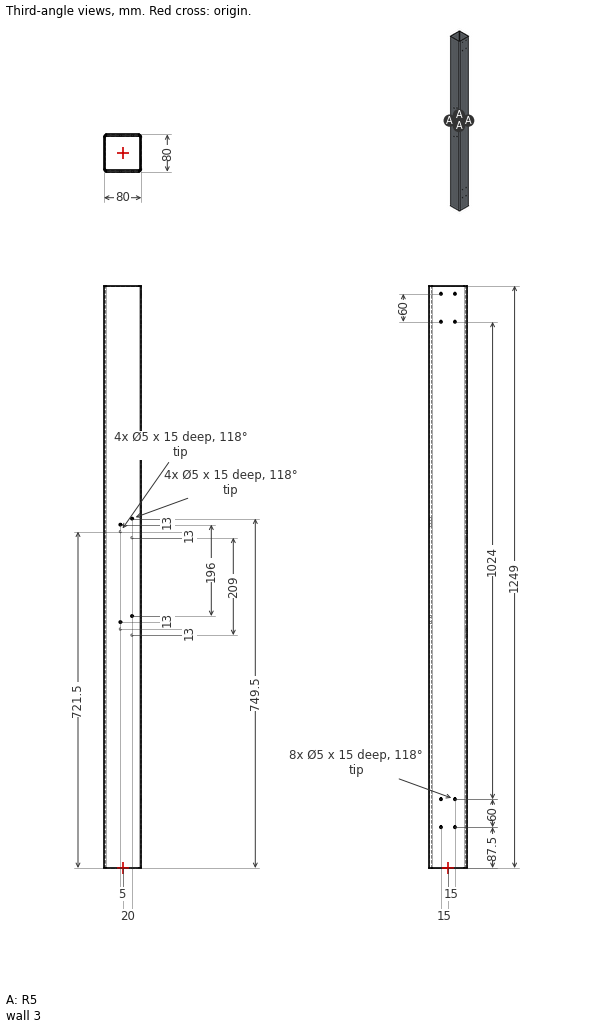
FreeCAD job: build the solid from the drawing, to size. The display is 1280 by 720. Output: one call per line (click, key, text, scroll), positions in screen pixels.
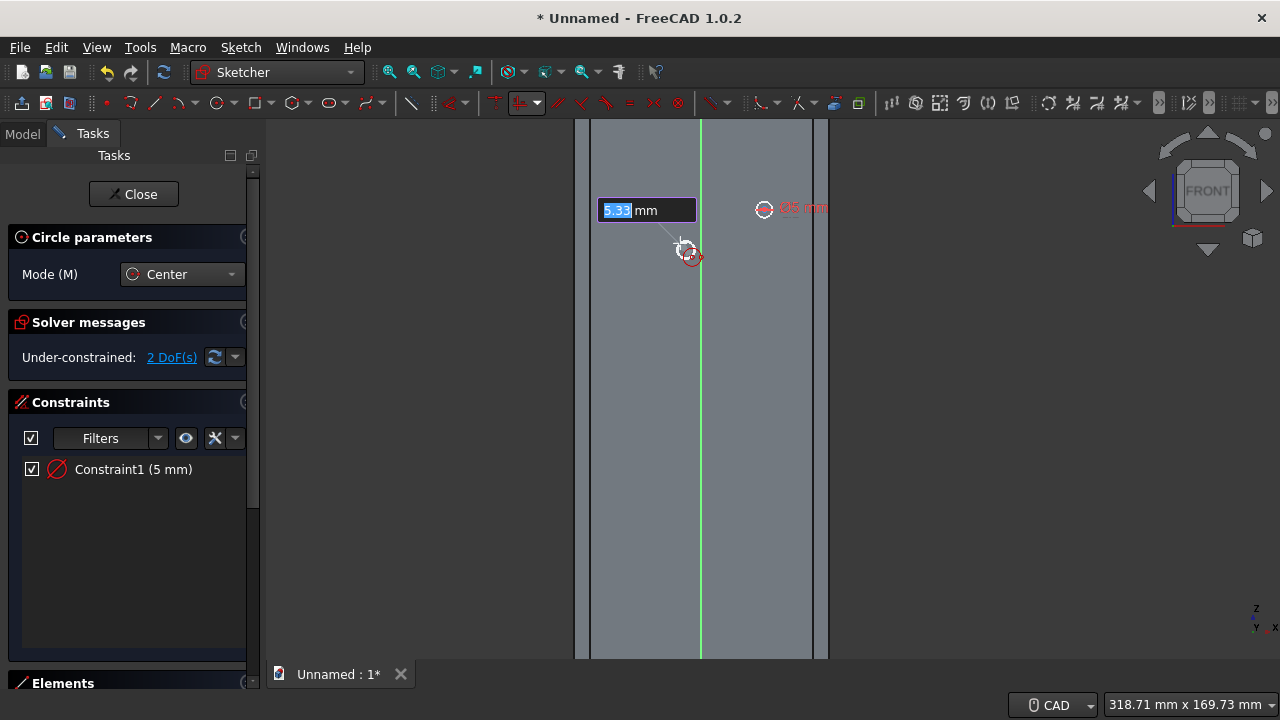
text(5)
key(Return)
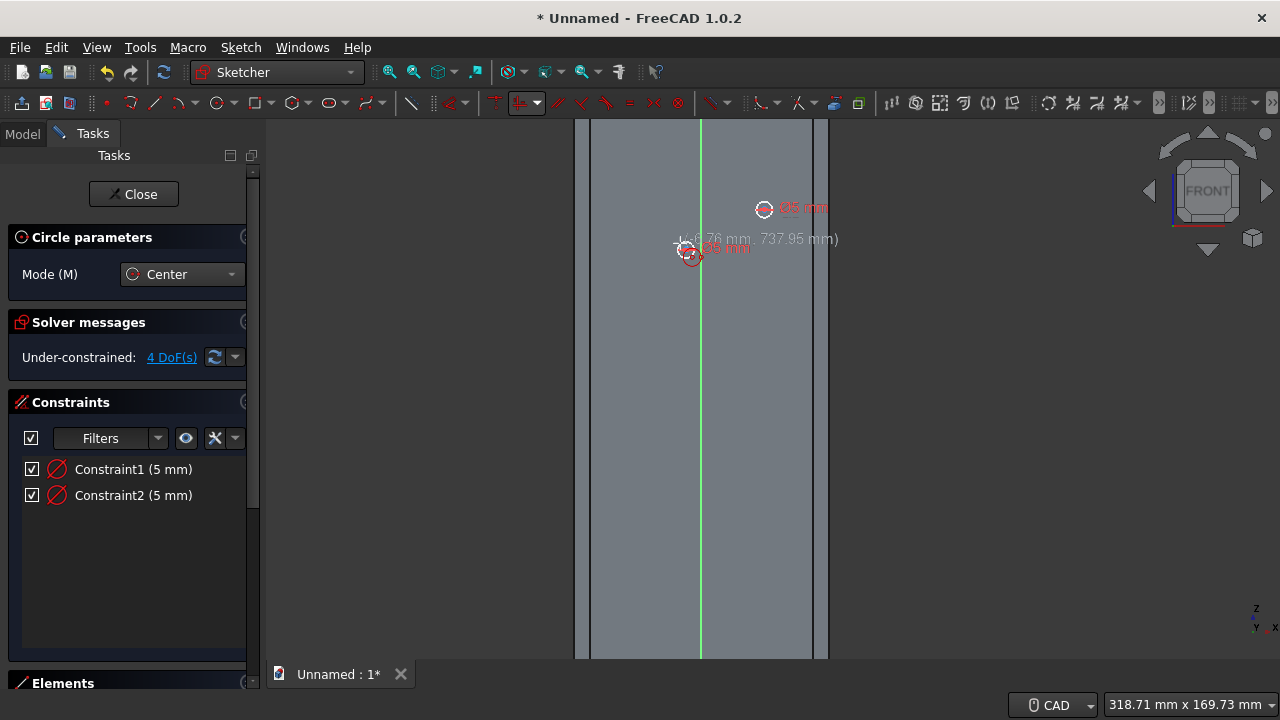
scroll(687, 249, down, 4)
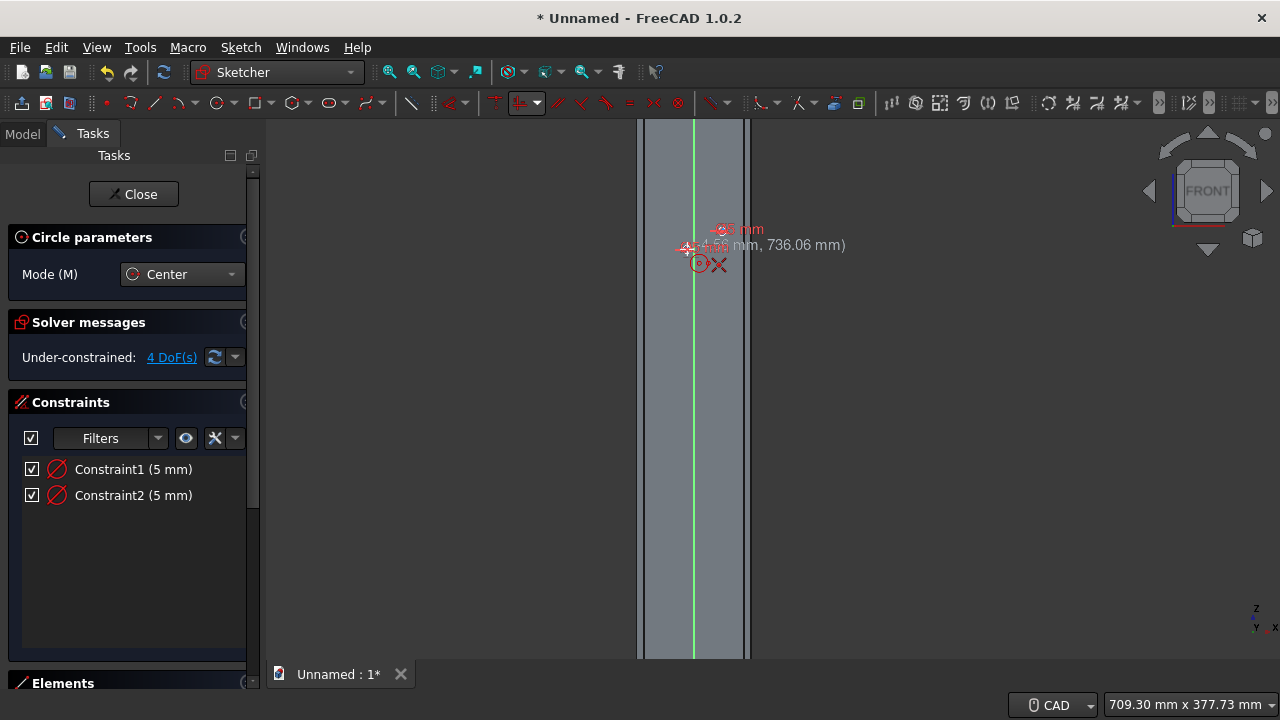
scroll(722, 529, up, 10)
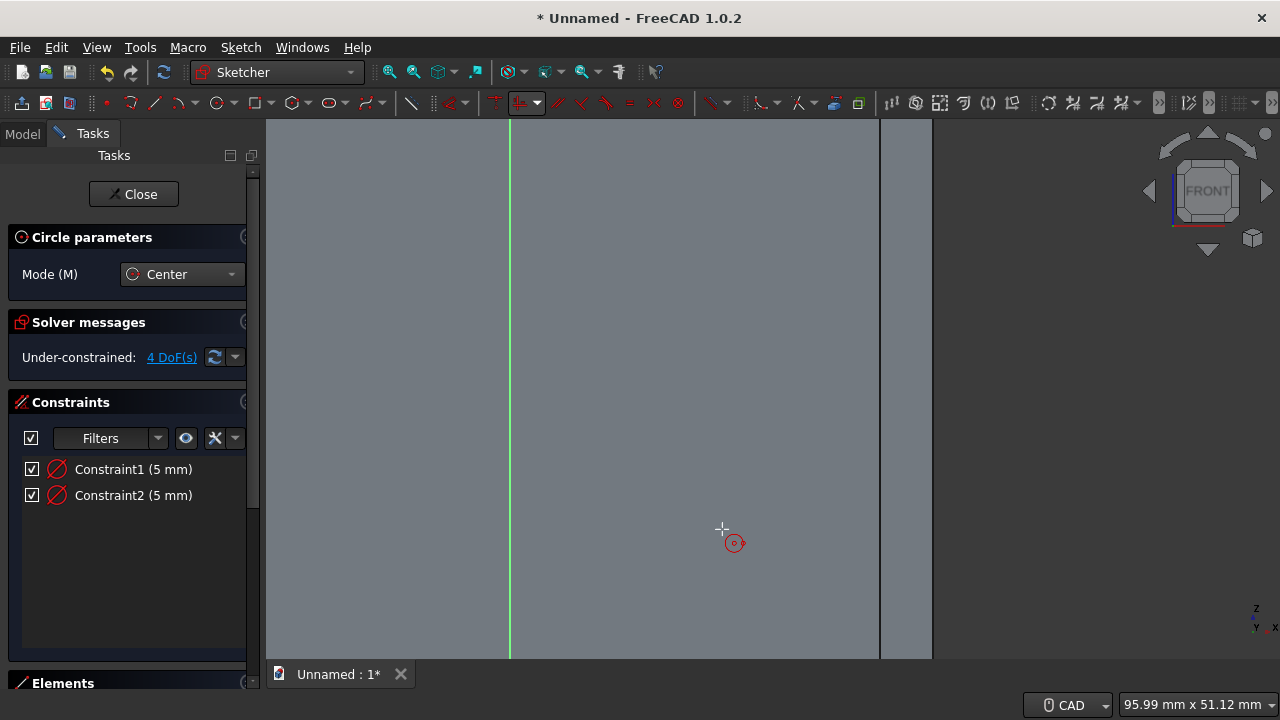
scroll(722, 530, down, 10)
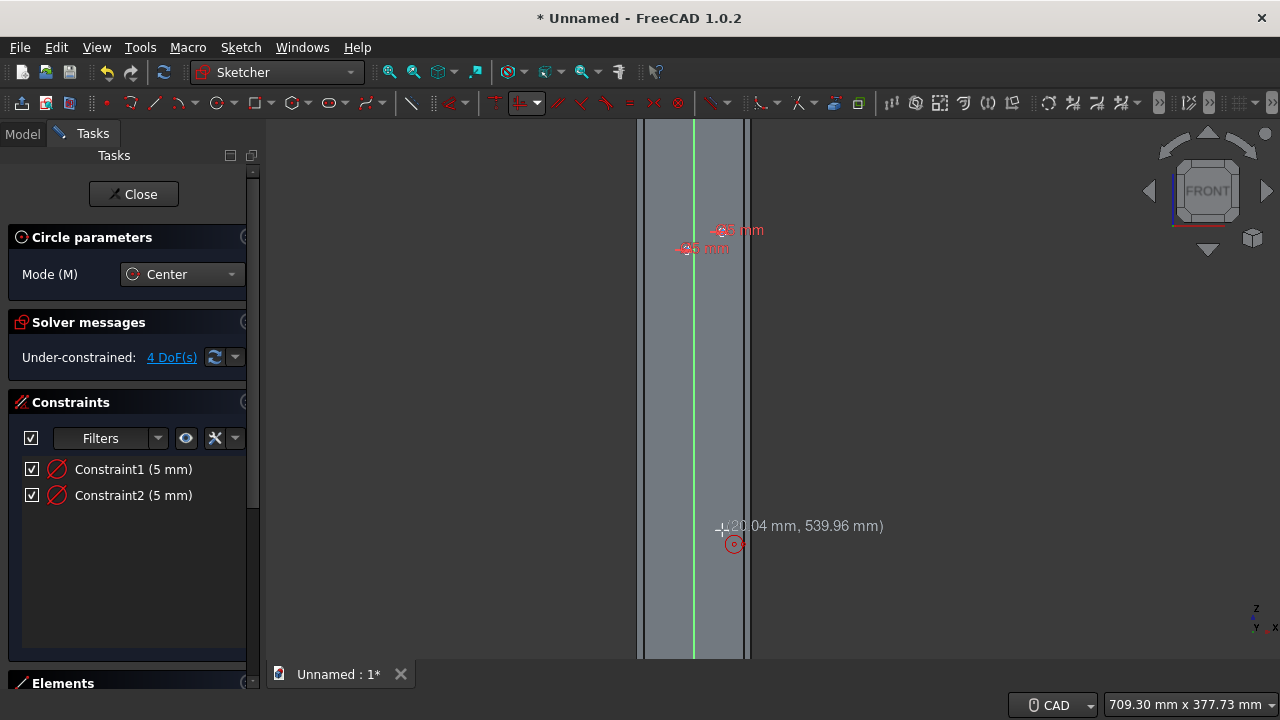
click(722, 530)
move(725, 527)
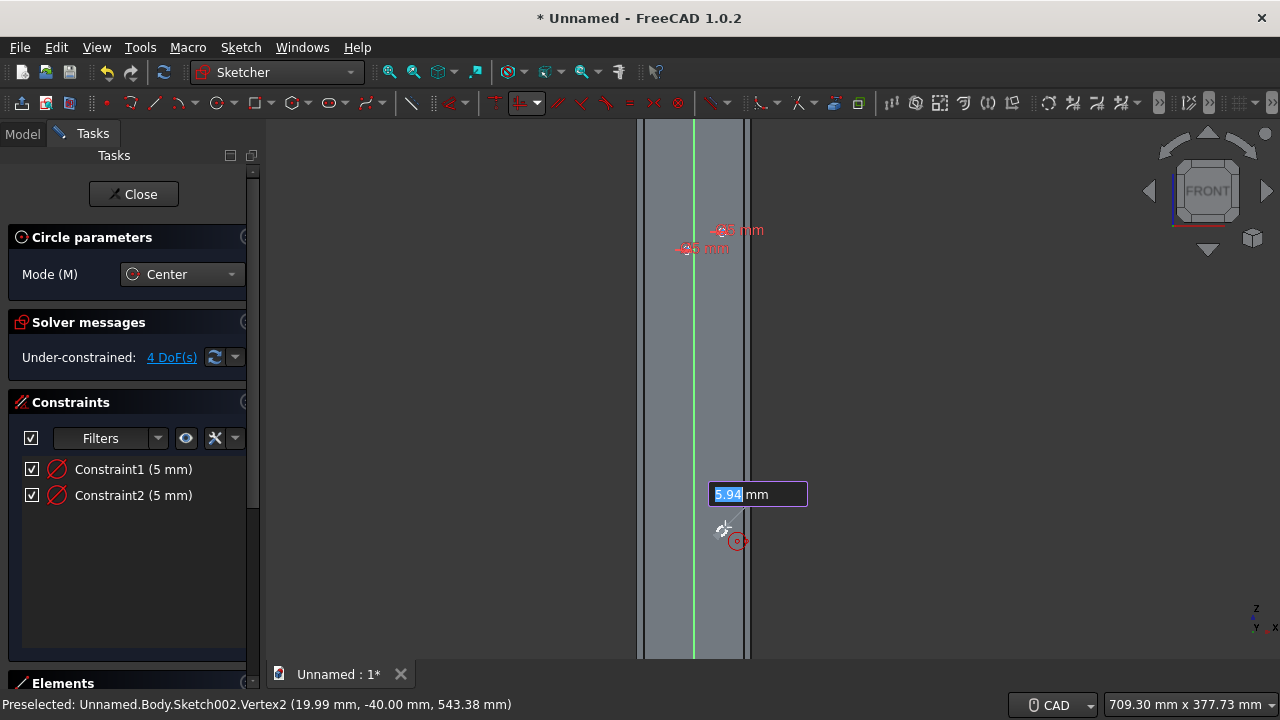
text(5)
key(Return)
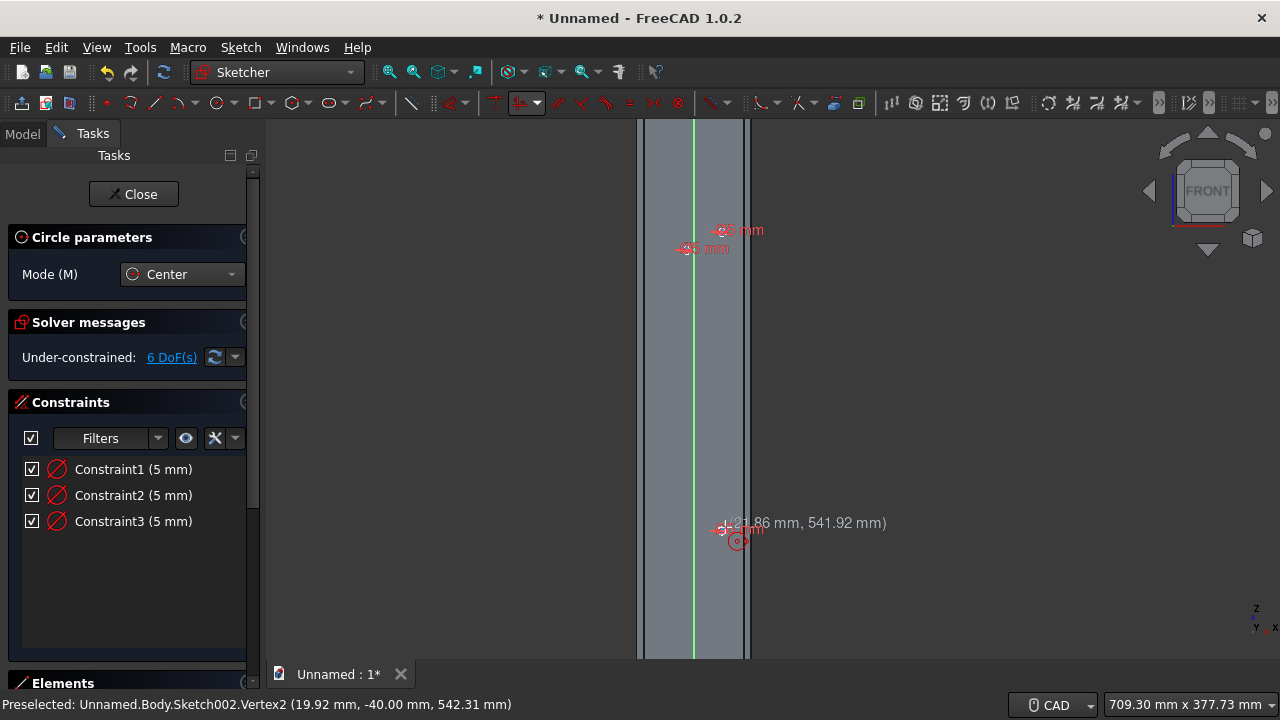
scroll(687, 549, up, 10)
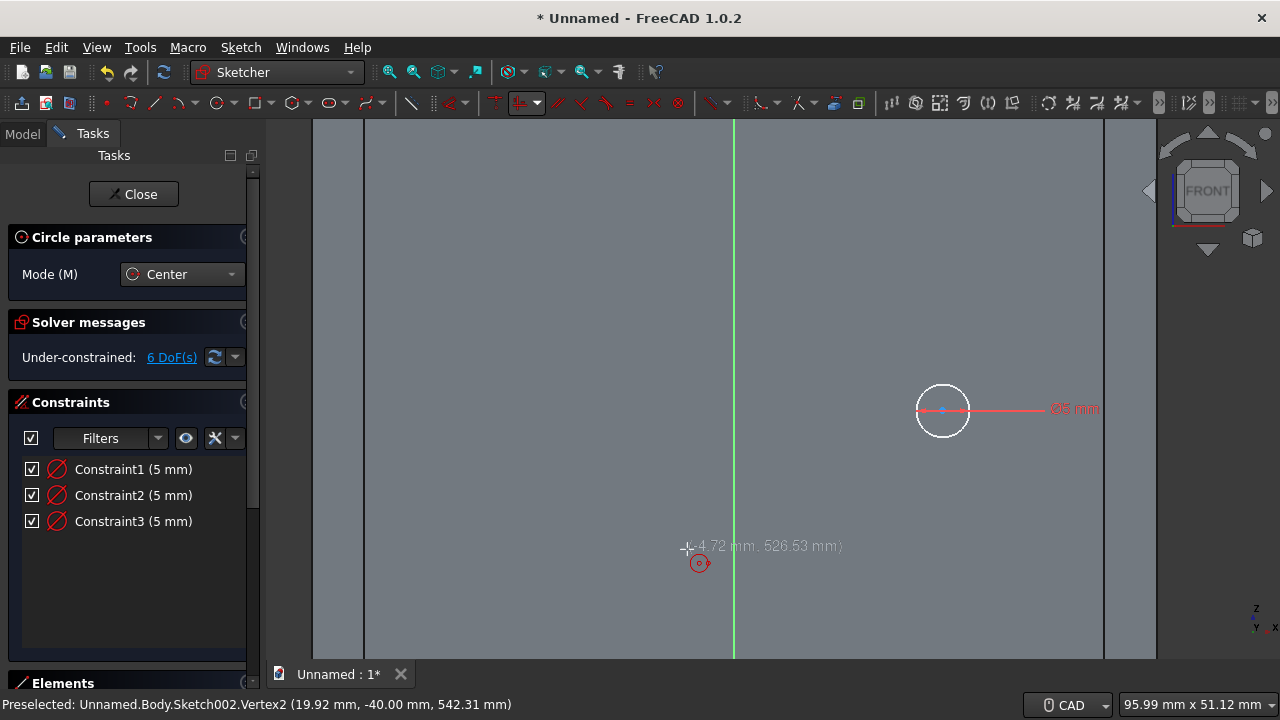
scroll(687, 549, down, 10)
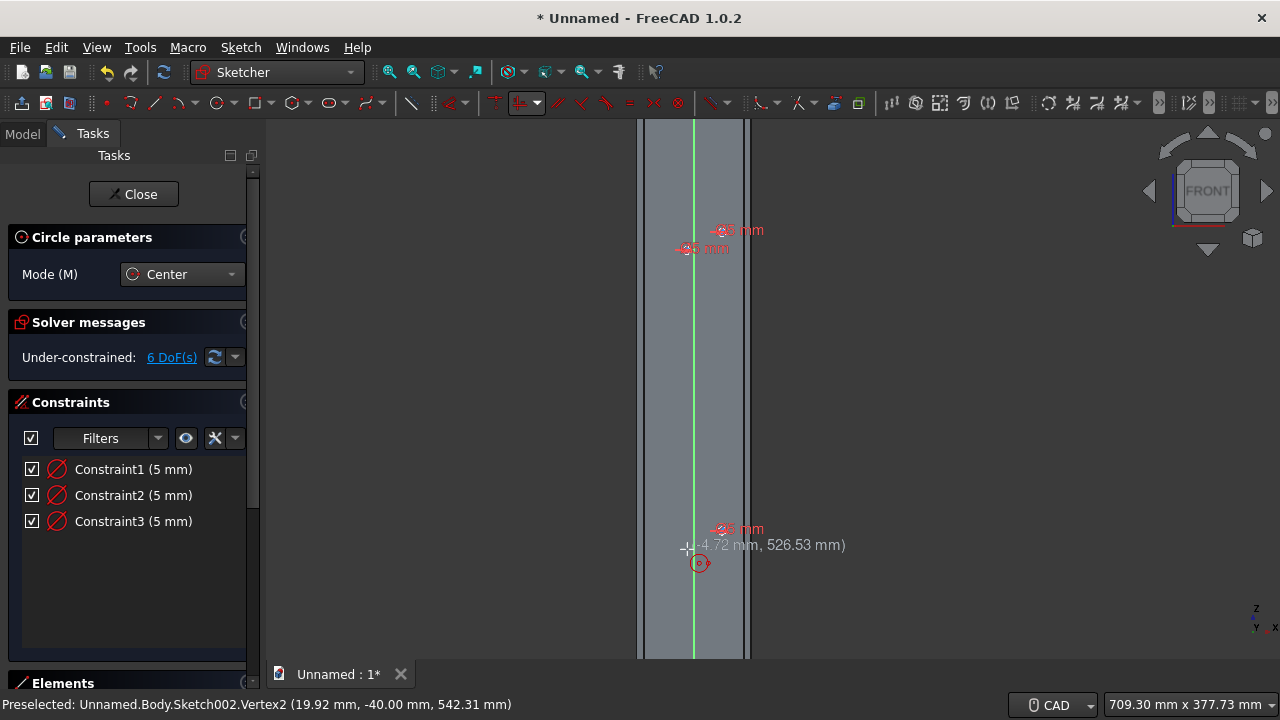
scroll(687, 549, up, 4)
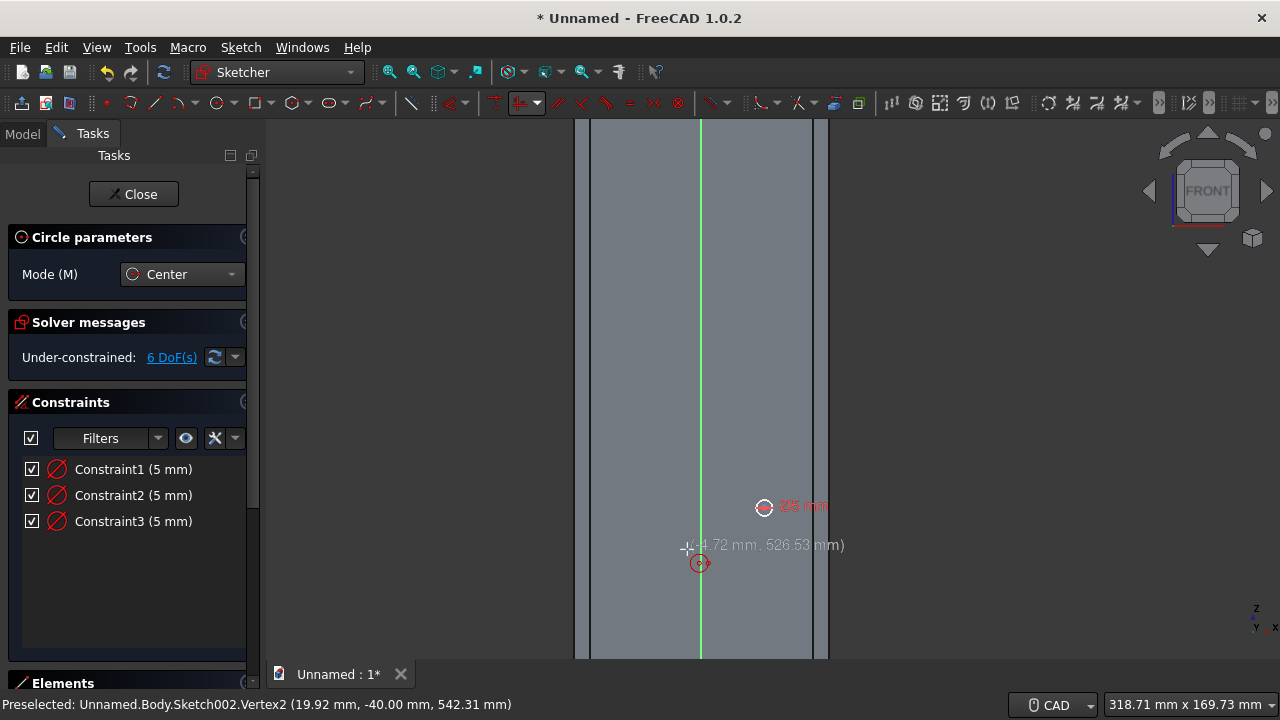
click(686, 547)
move(680, 542)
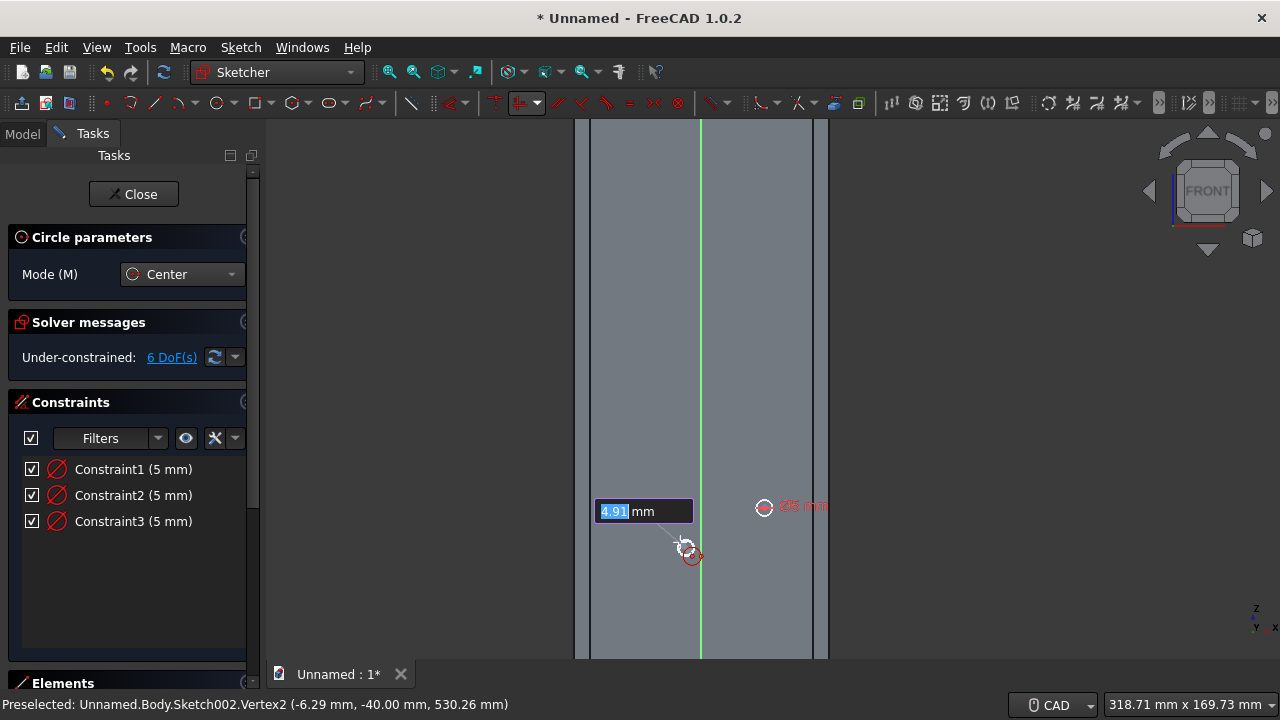
text(5)
key(Return)
key(Escape)